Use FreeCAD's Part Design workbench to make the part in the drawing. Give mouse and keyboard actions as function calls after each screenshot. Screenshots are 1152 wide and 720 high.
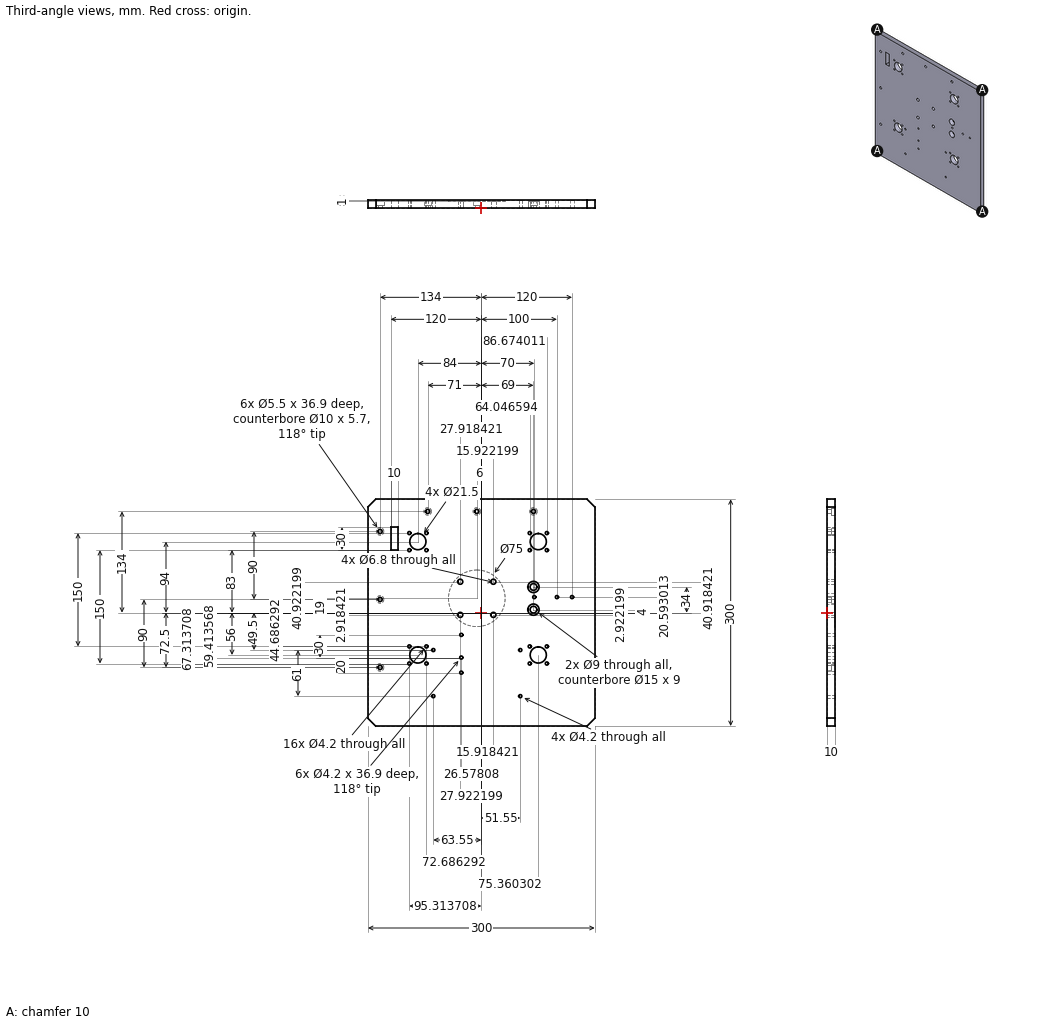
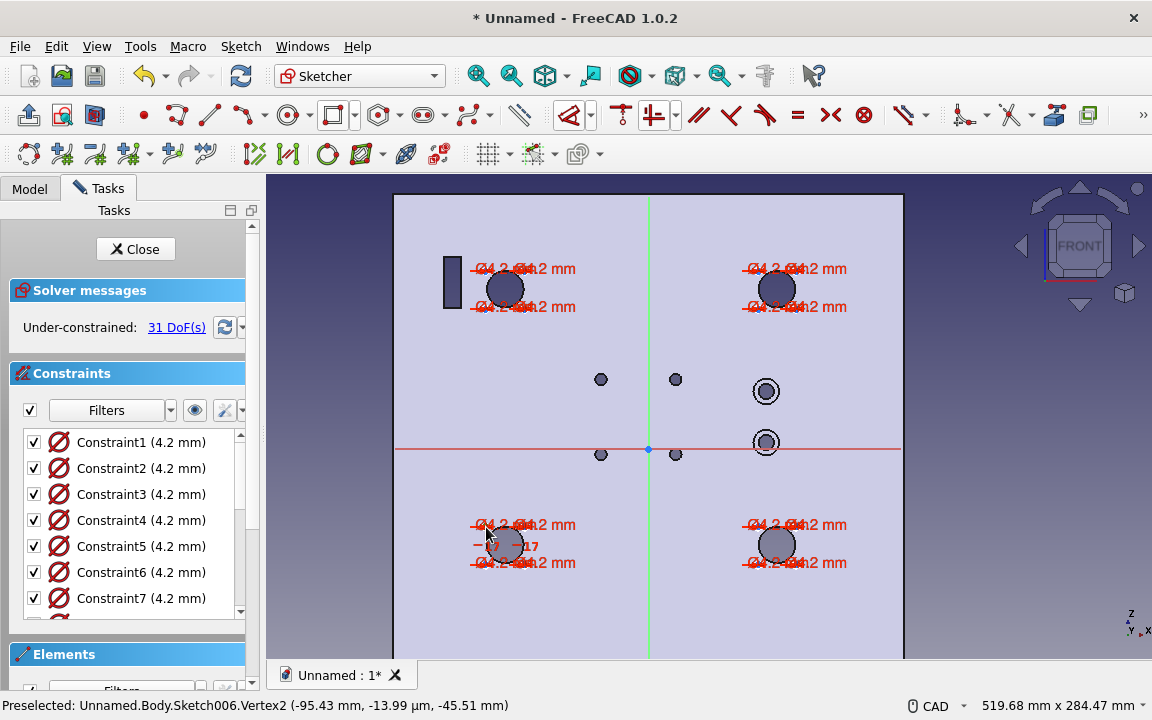
click(486, 565)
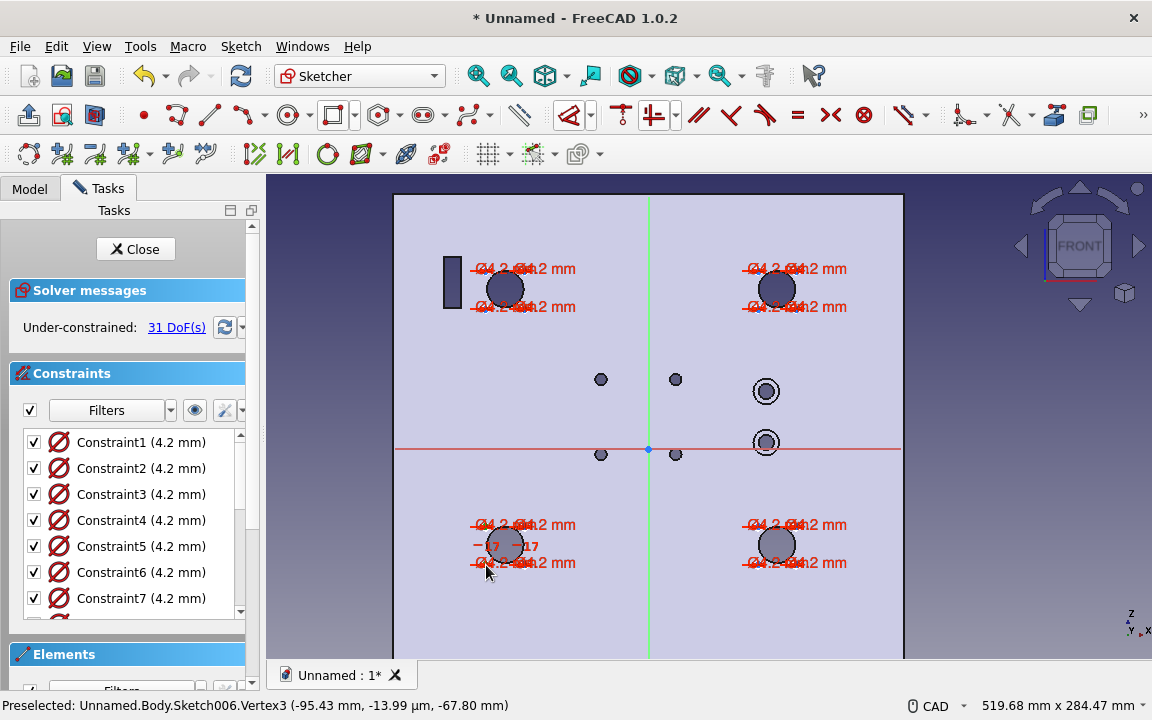
key(v)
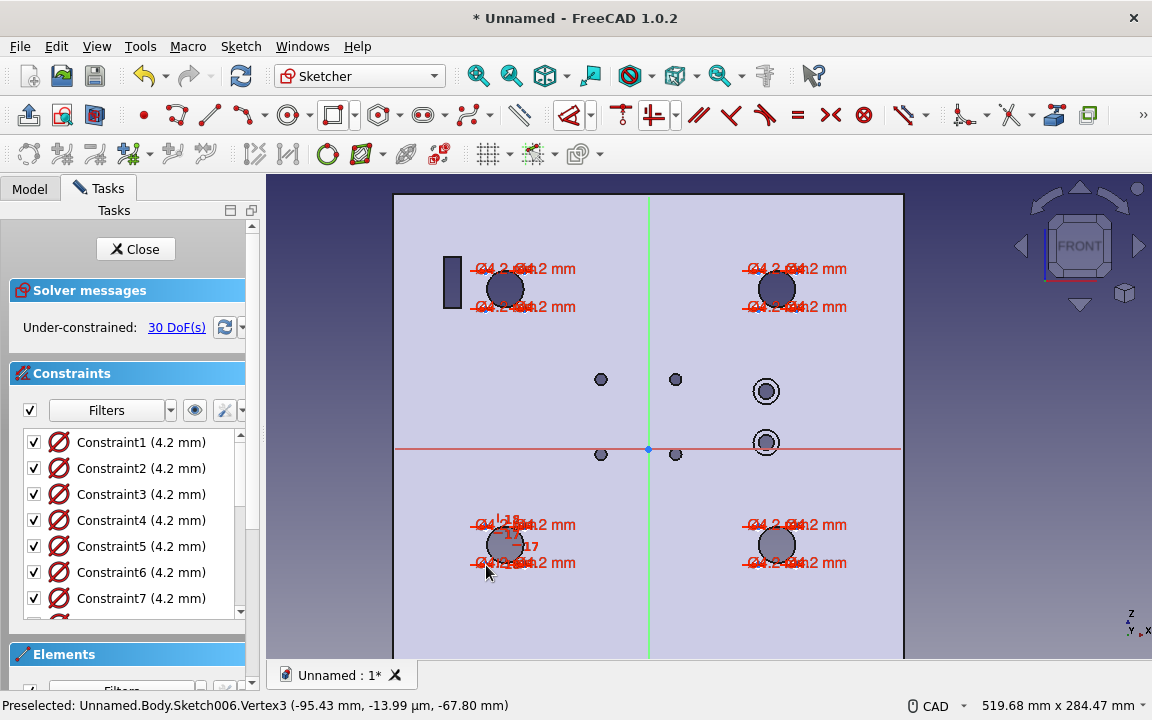
click(525, 527)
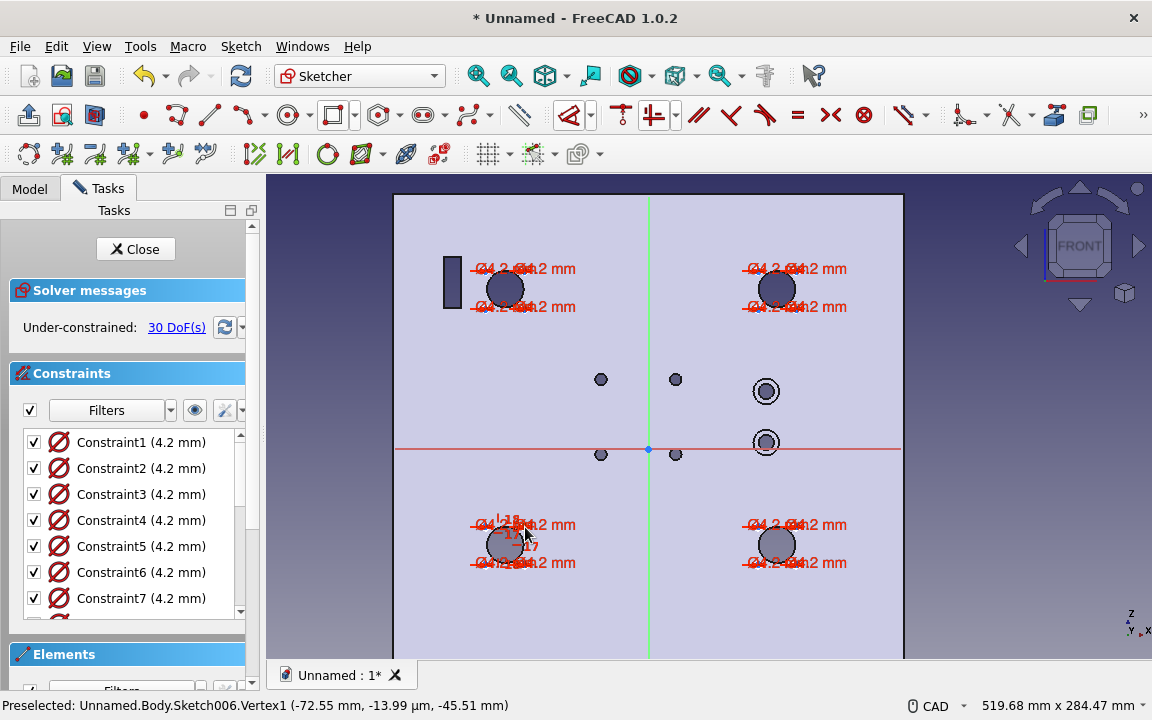
click(525, 565)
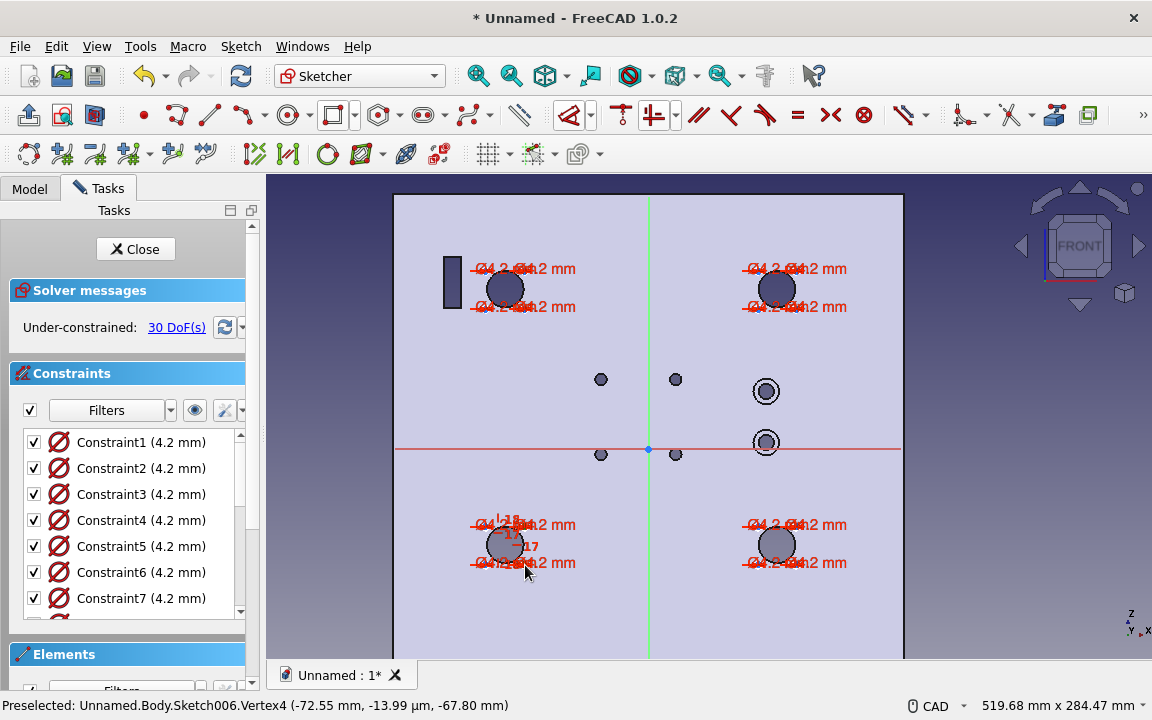
click(676, 116)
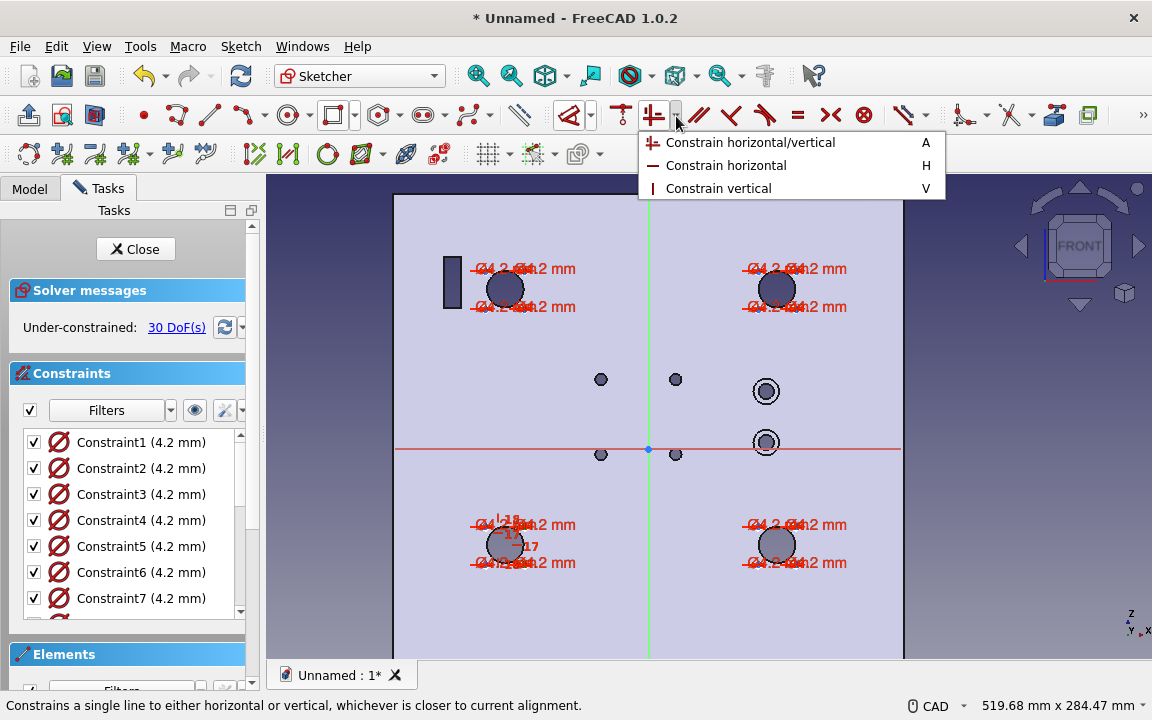
click(792, 188)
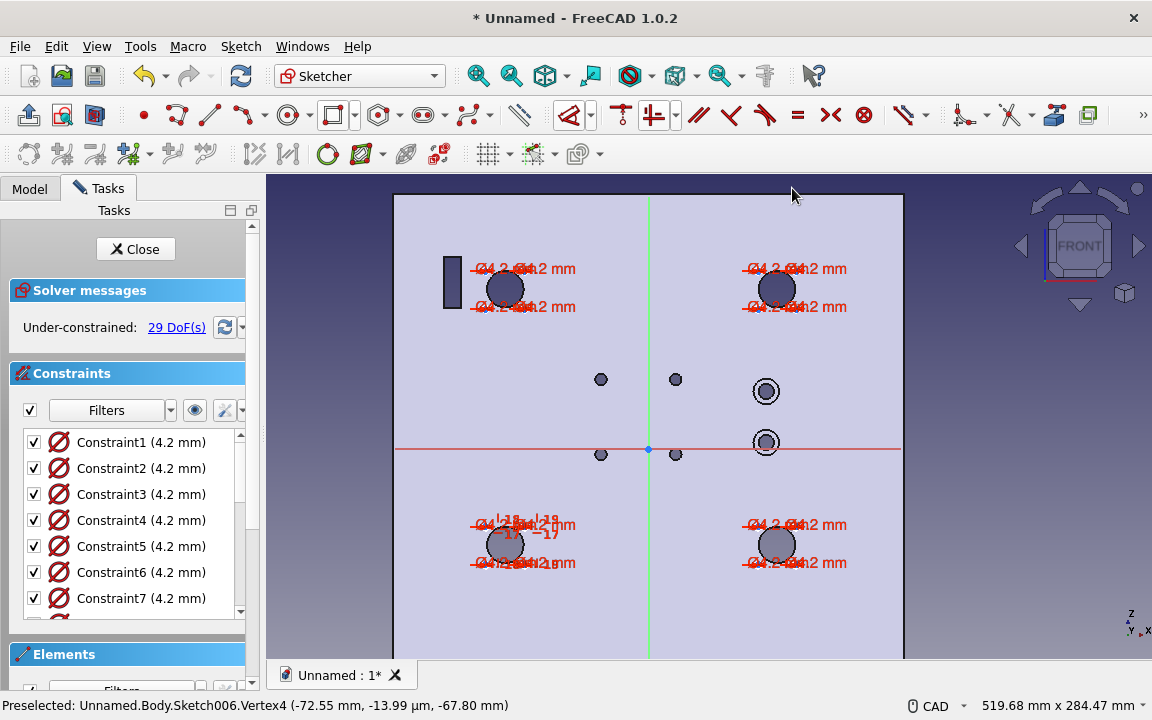
click(486, 565)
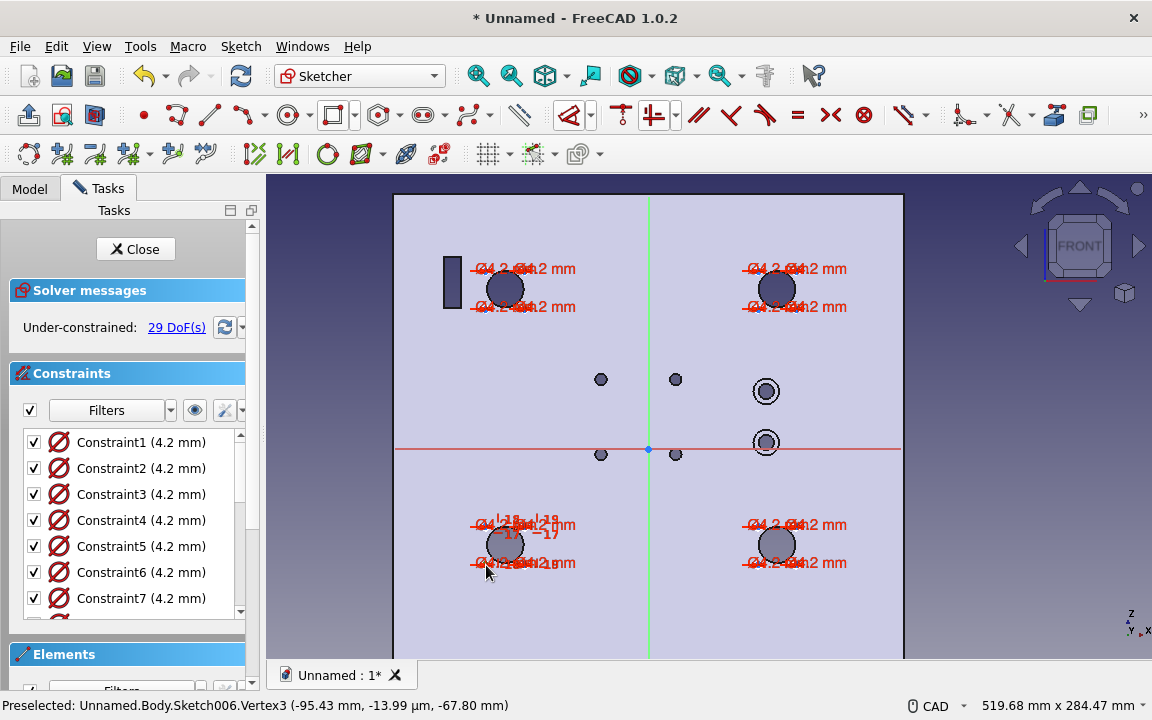
click(525, 565)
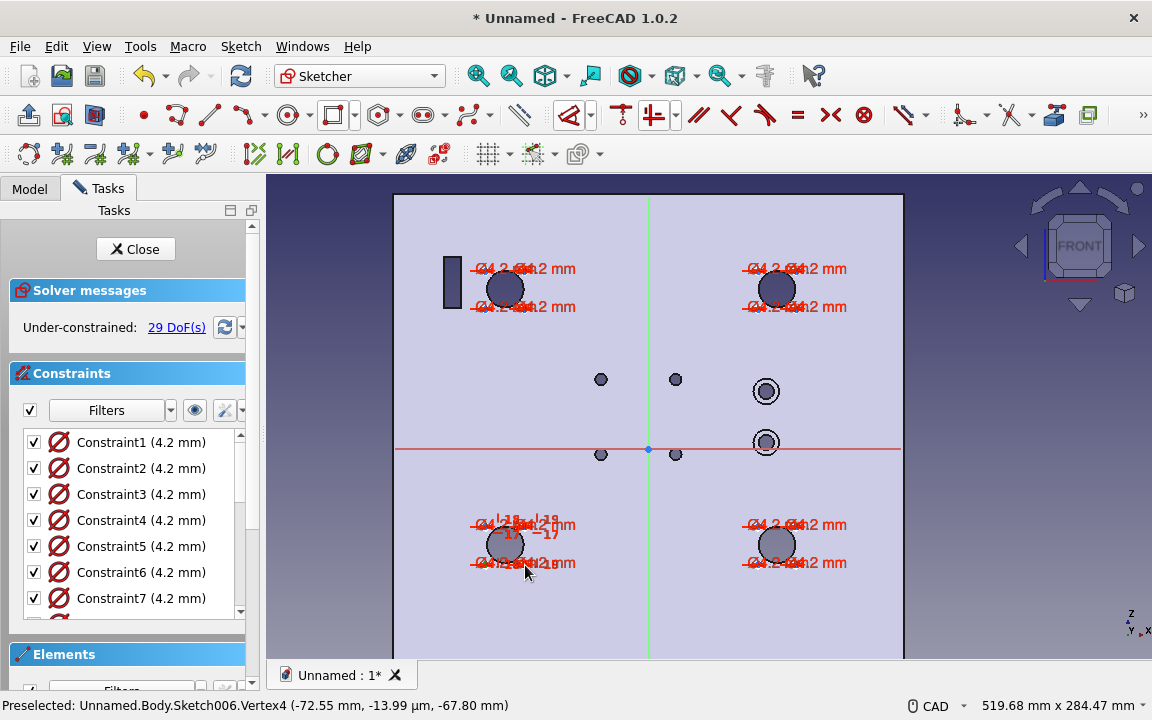
key(h)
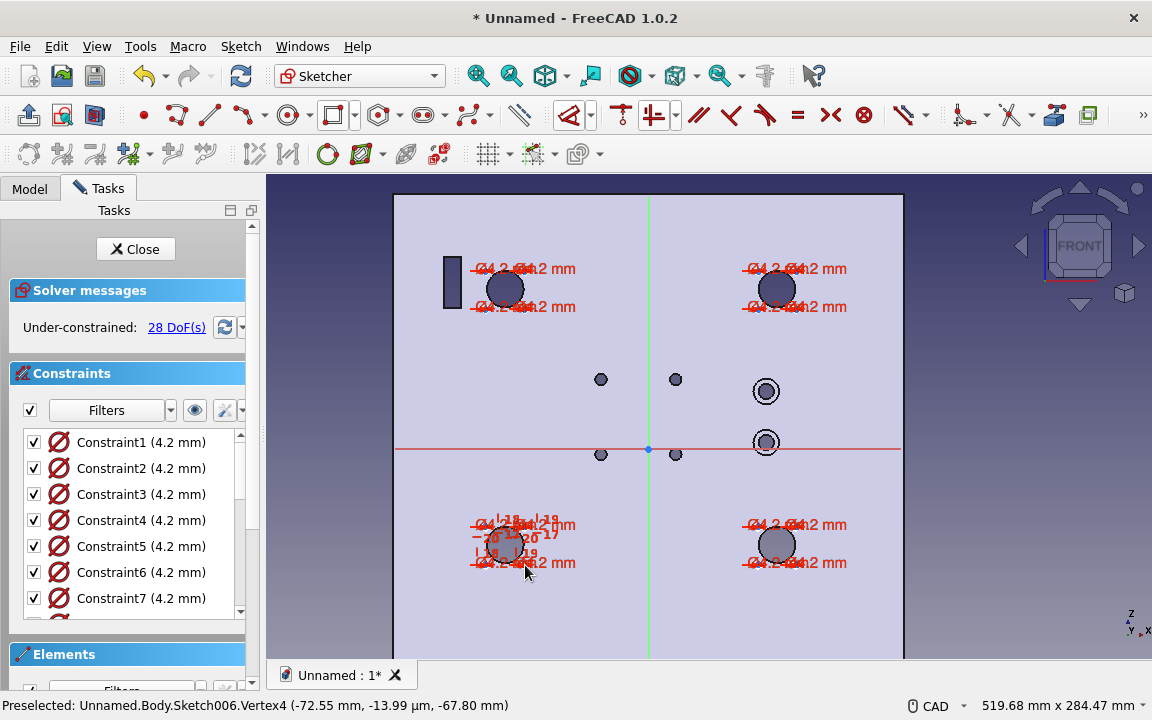
click(486, 527)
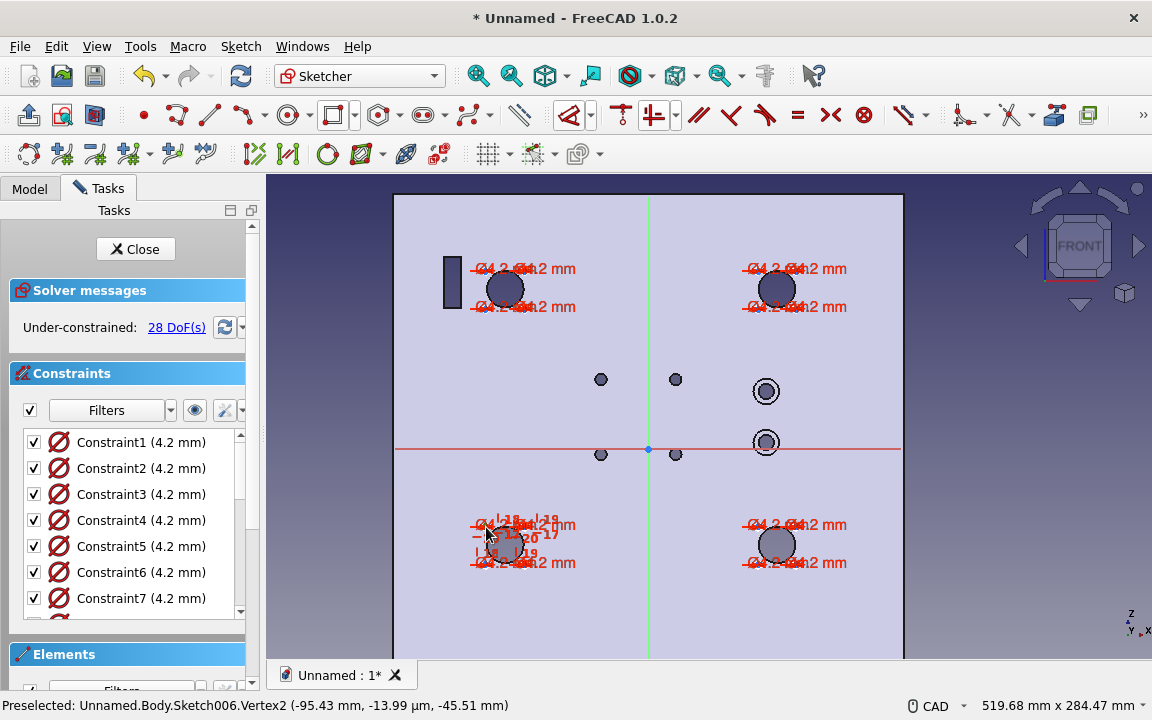
click(486, 309)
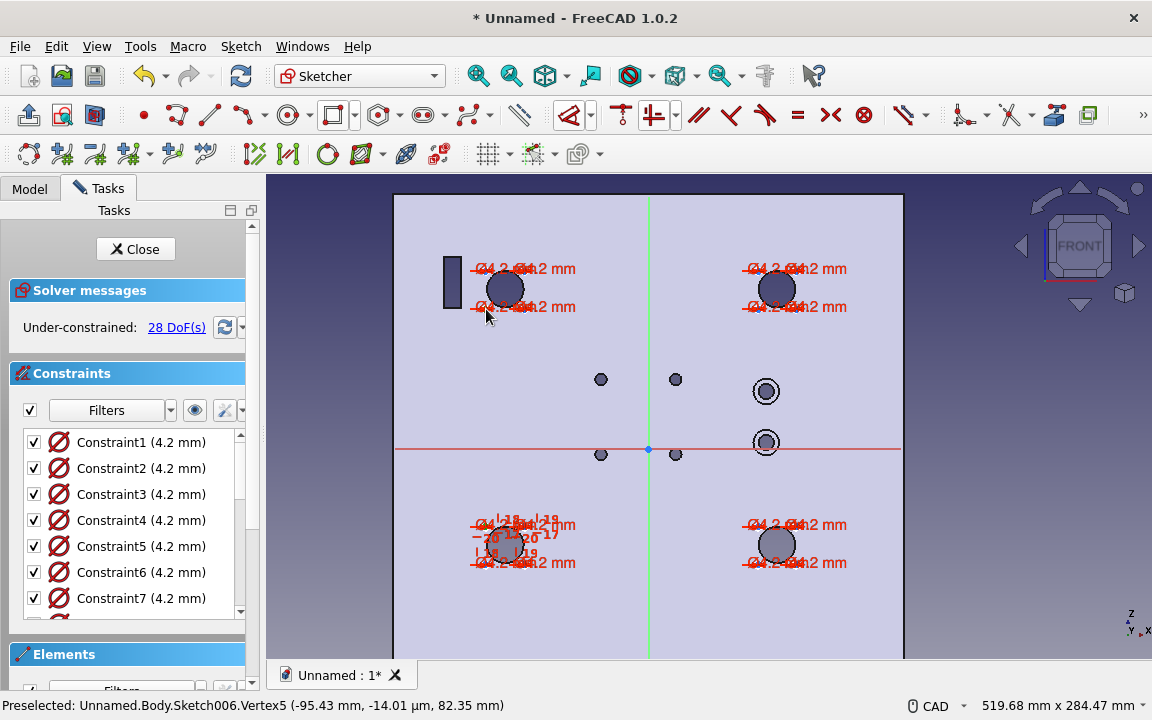
key(v)